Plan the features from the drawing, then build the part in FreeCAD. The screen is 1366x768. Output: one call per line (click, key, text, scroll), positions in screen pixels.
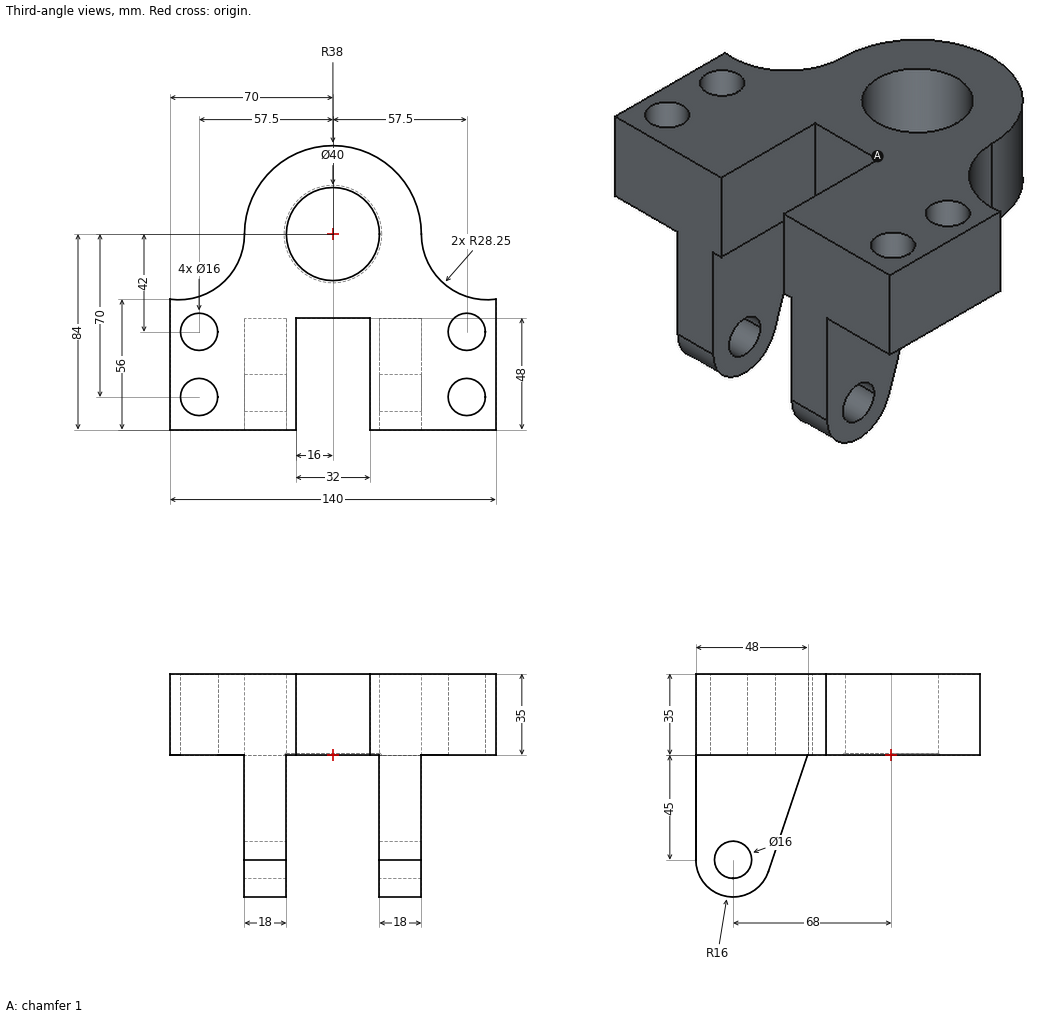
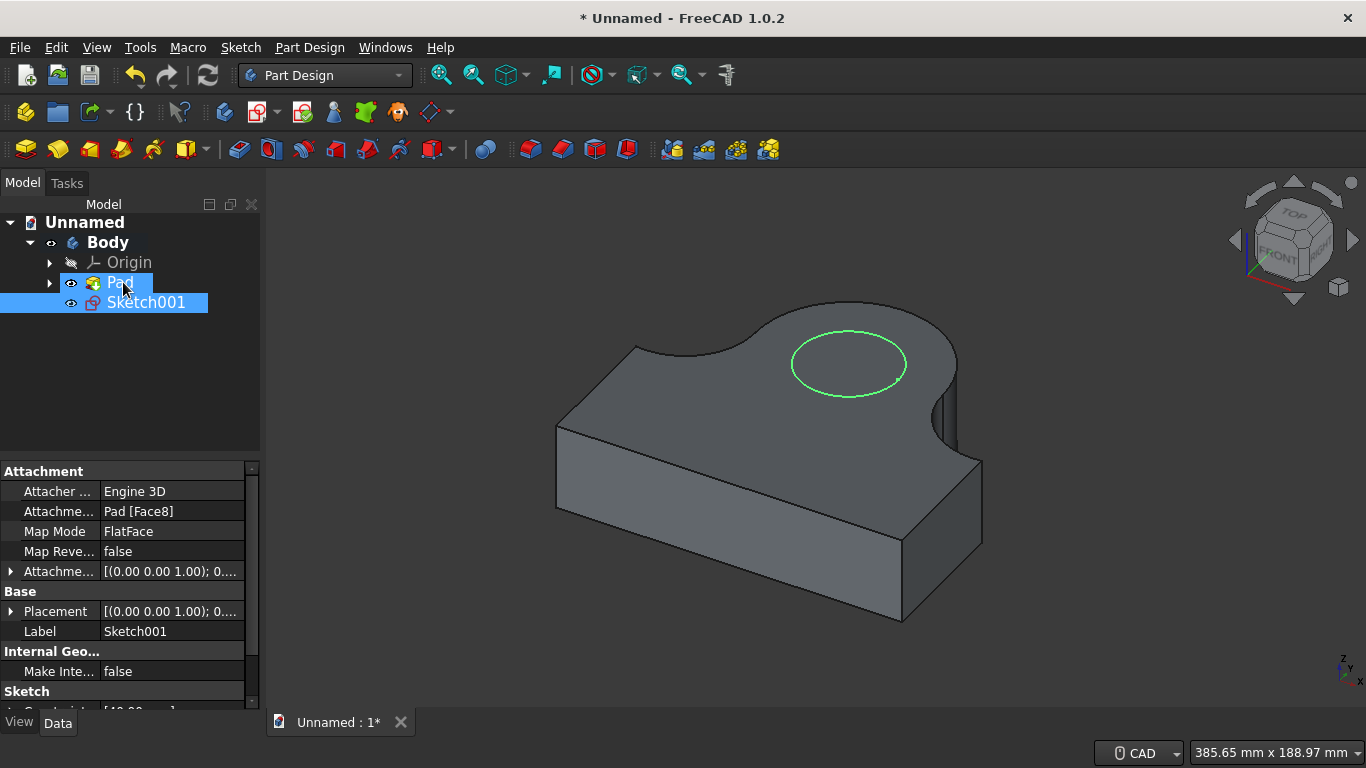
click(240, 150)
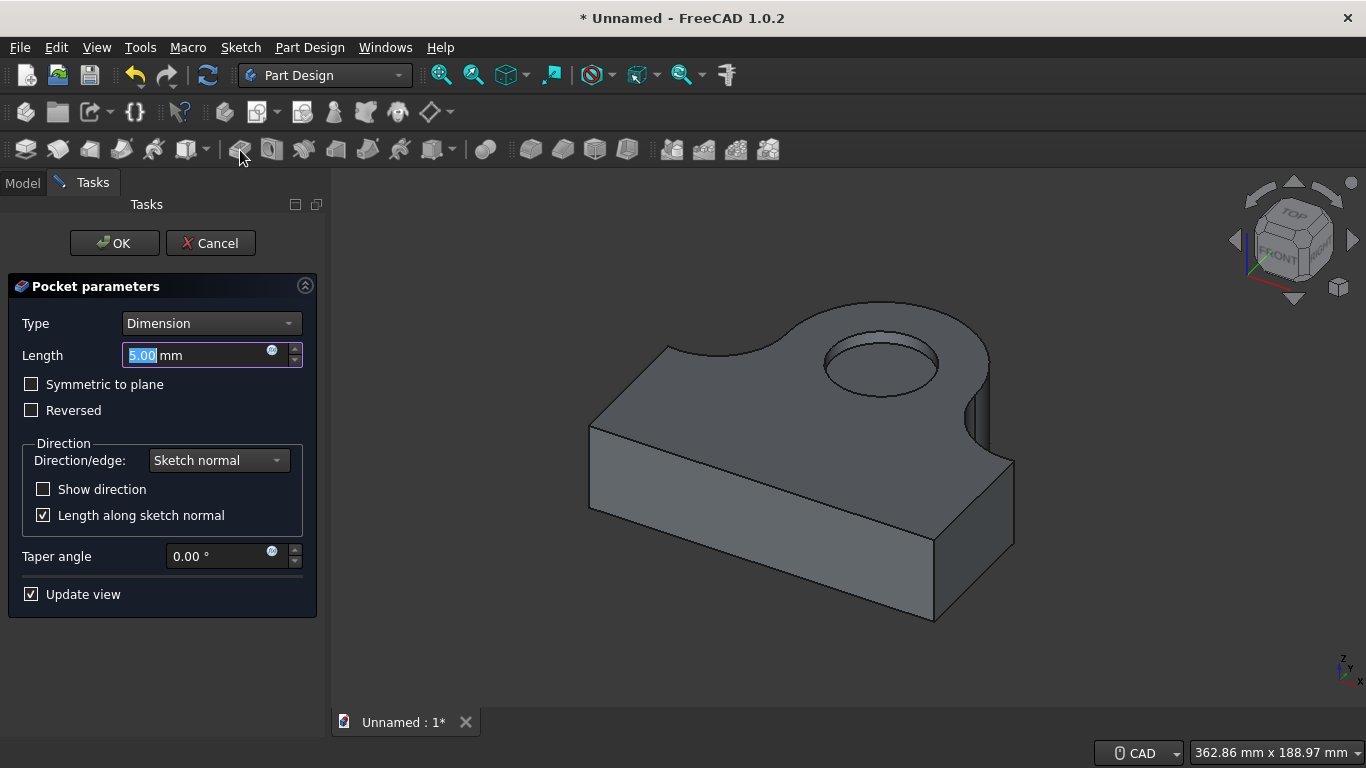
text(35)
key(Tab)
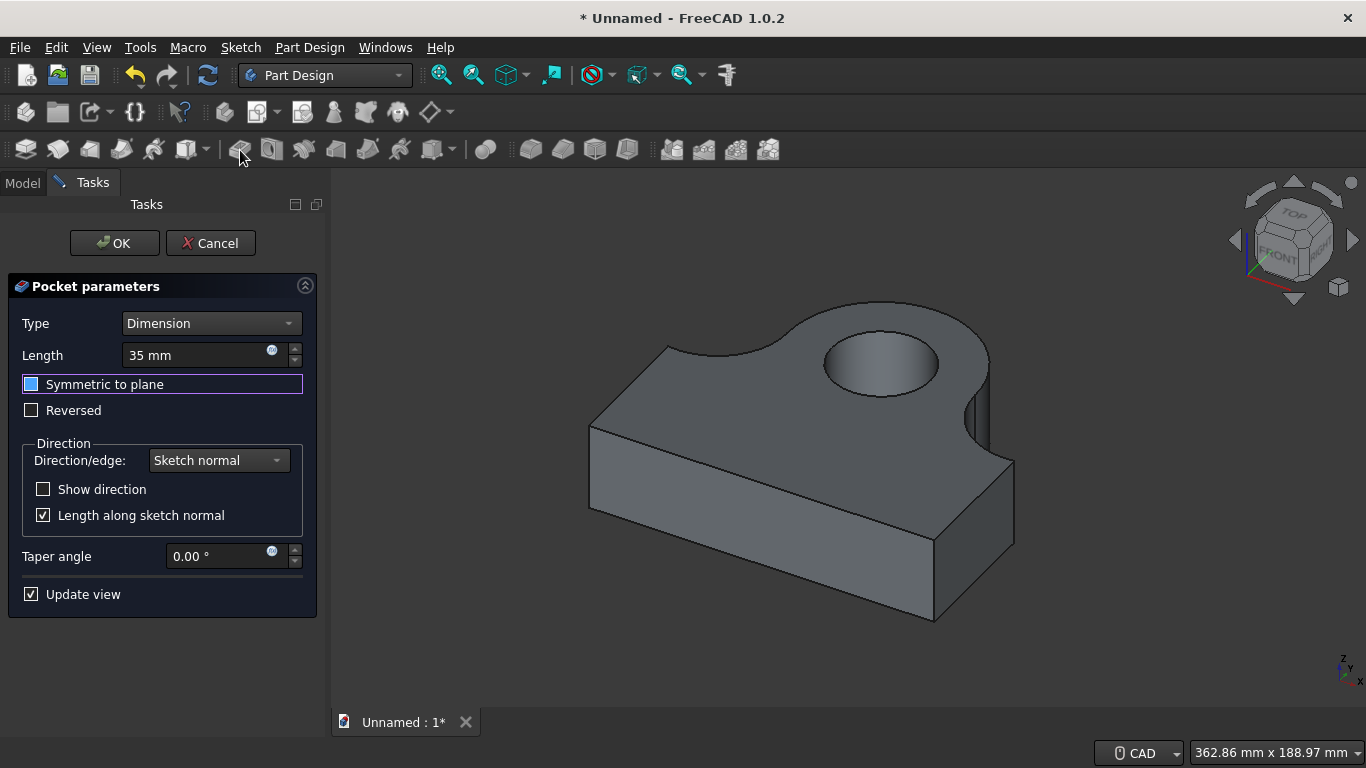
click(115, 243)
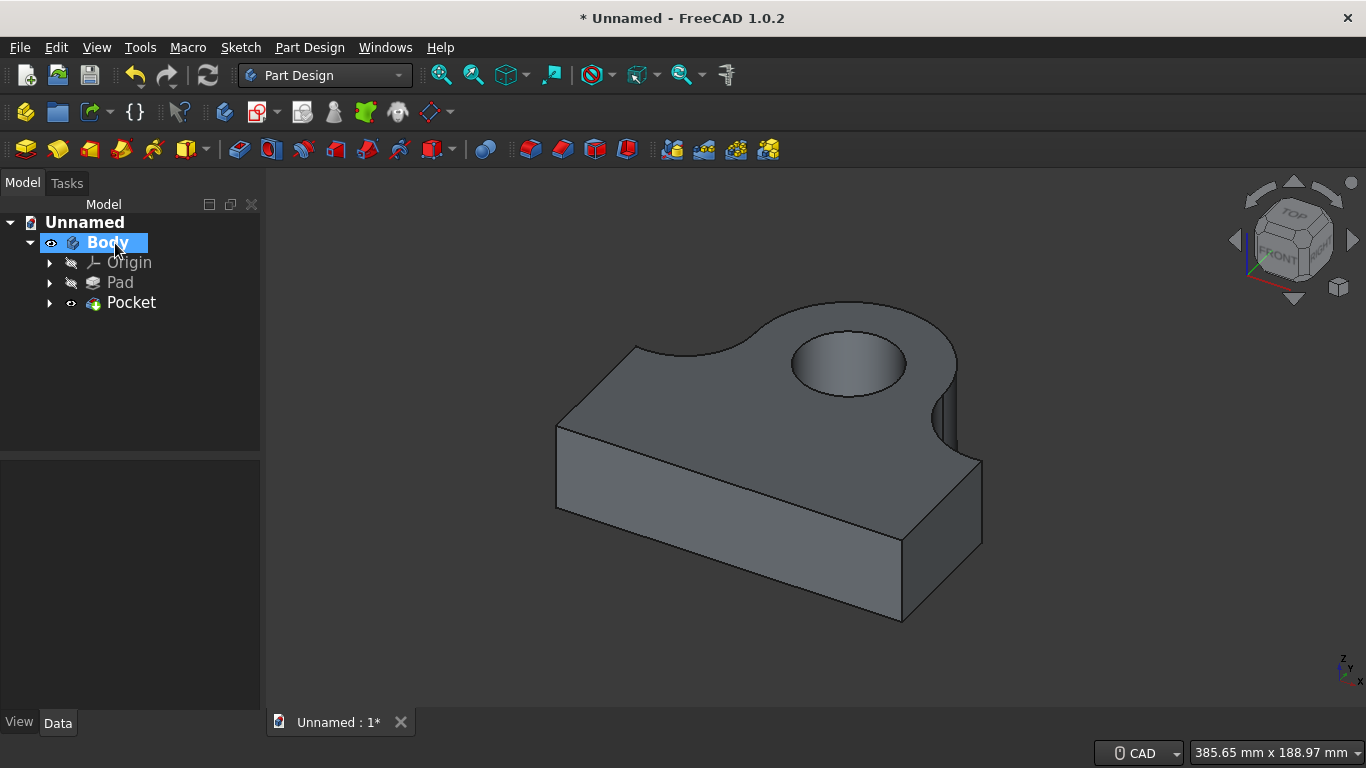
click(865, 478)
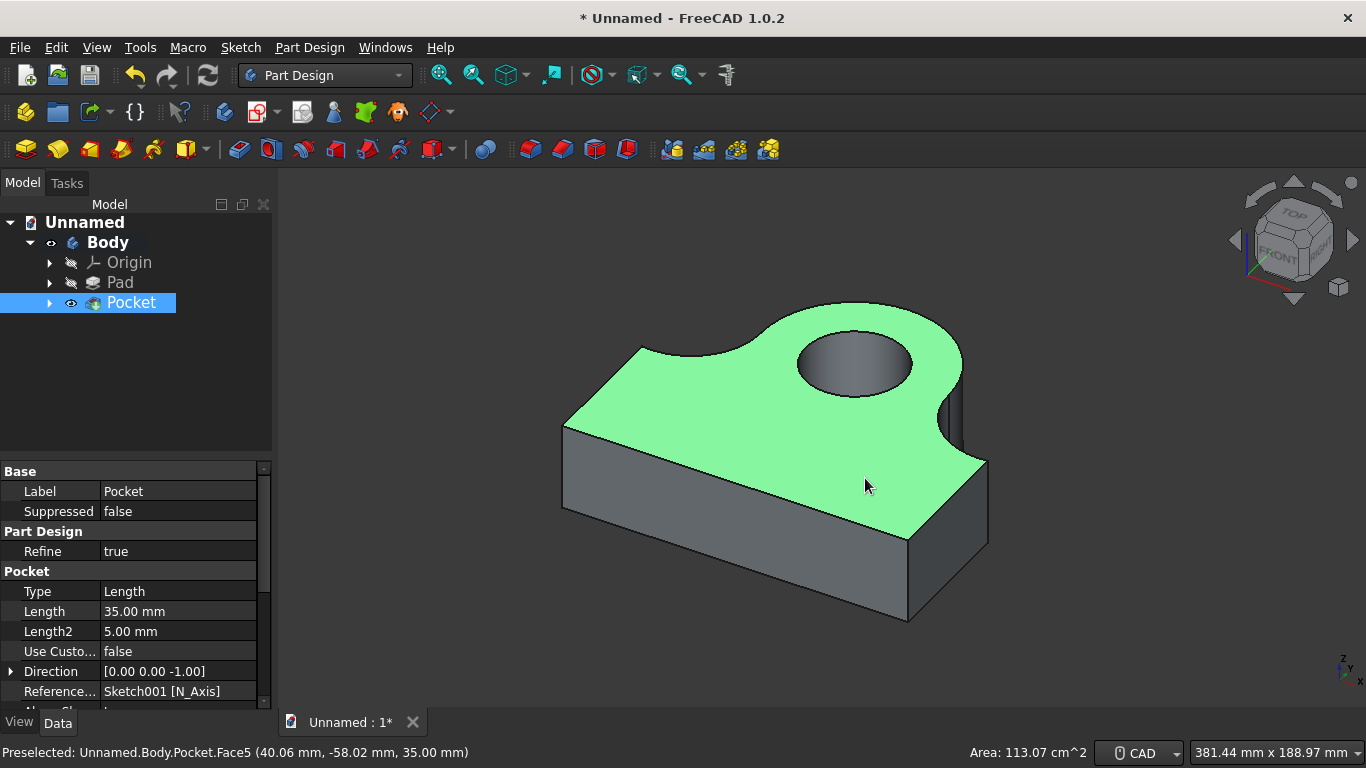
click(258, 112)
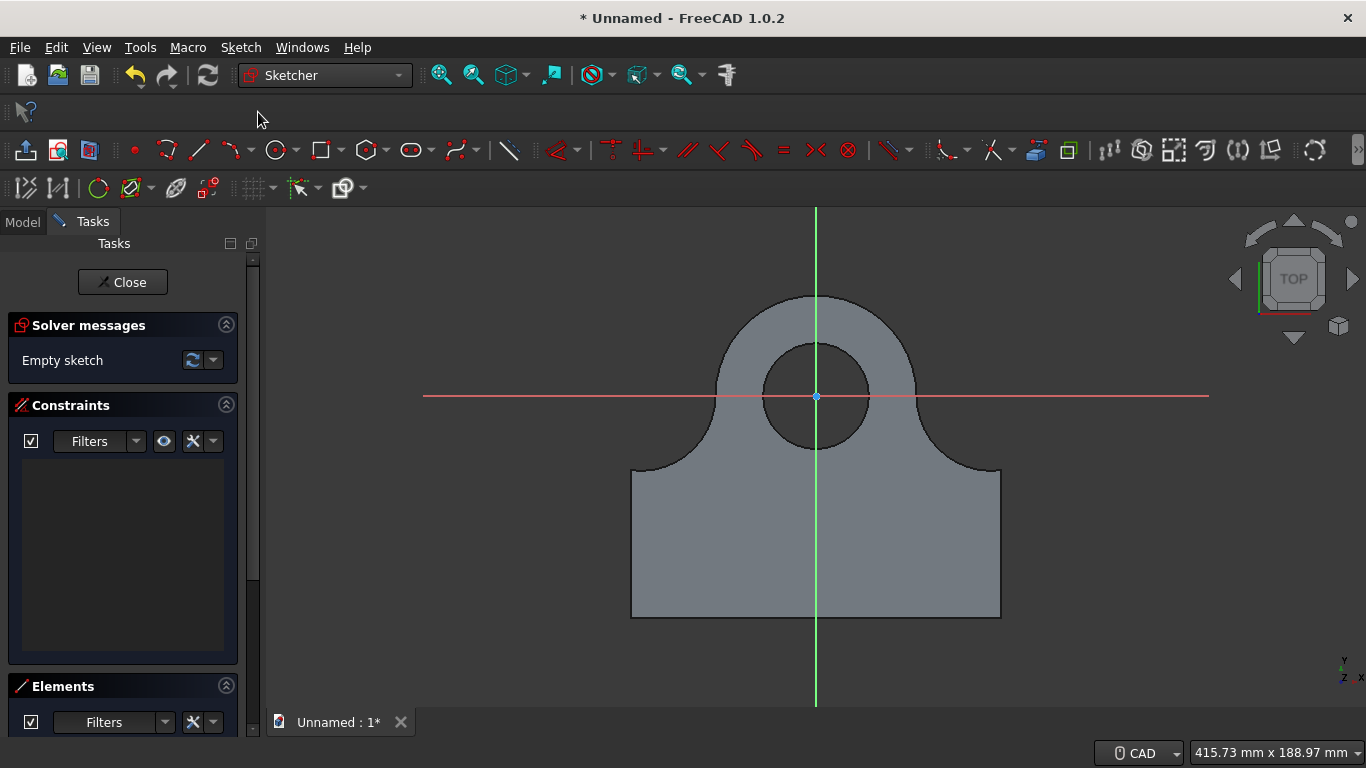
scroll(955, 585, up, 2)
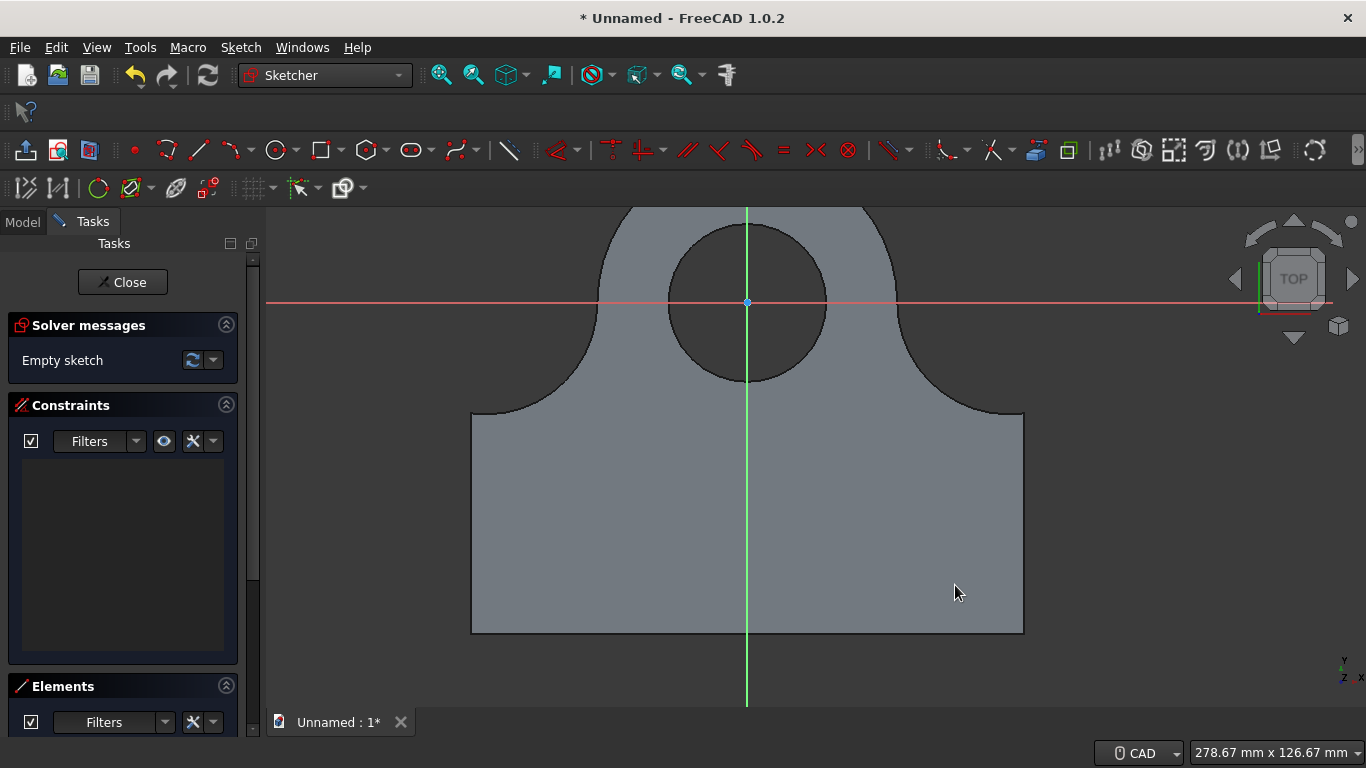
click(276, 150)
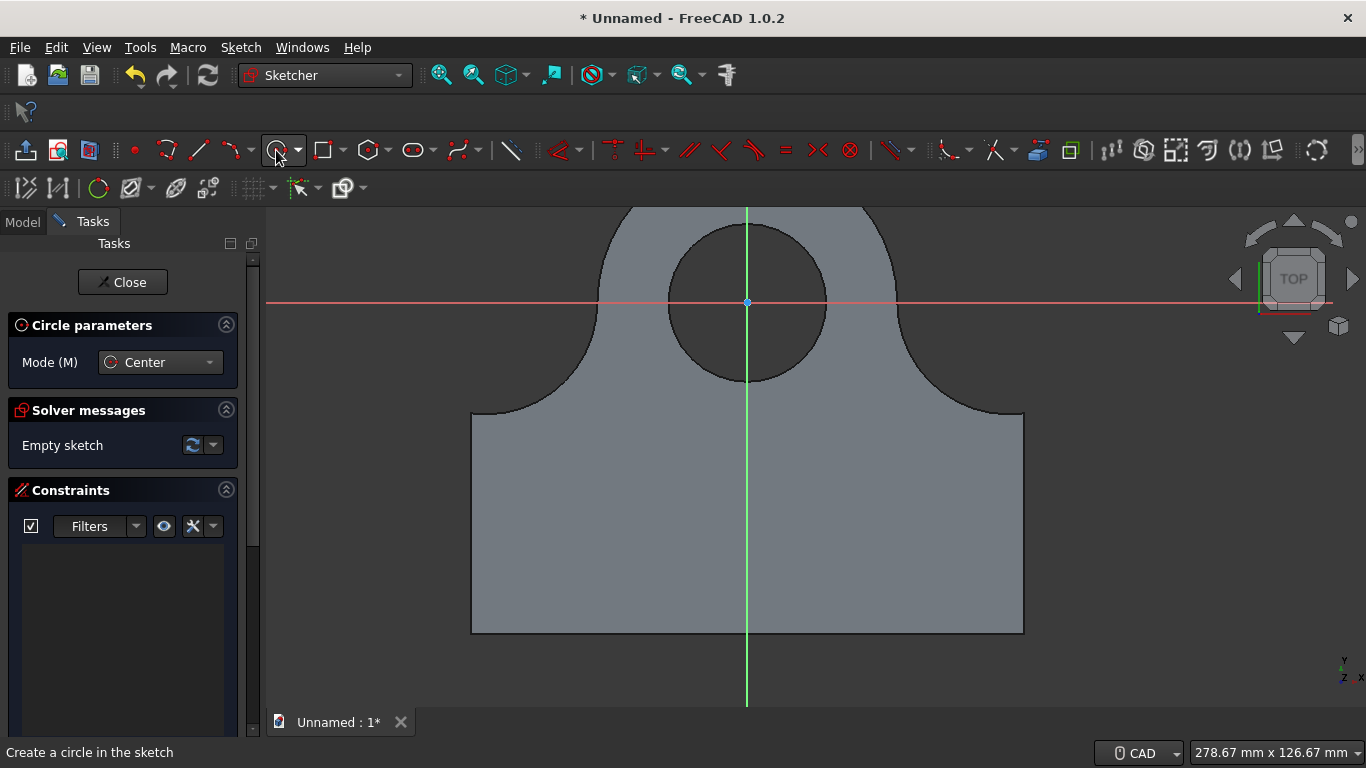
click(520, 469)
move(543, 446)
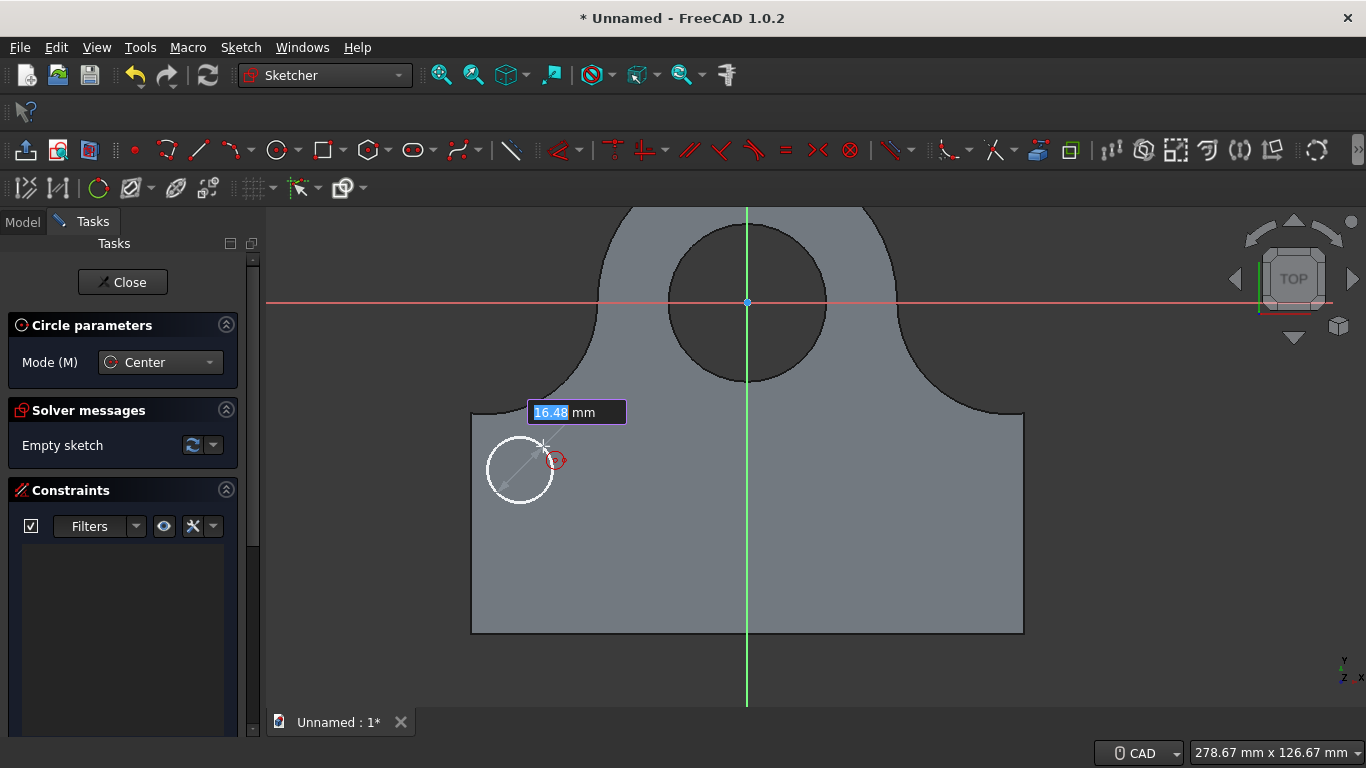
text(16)
key(Return)